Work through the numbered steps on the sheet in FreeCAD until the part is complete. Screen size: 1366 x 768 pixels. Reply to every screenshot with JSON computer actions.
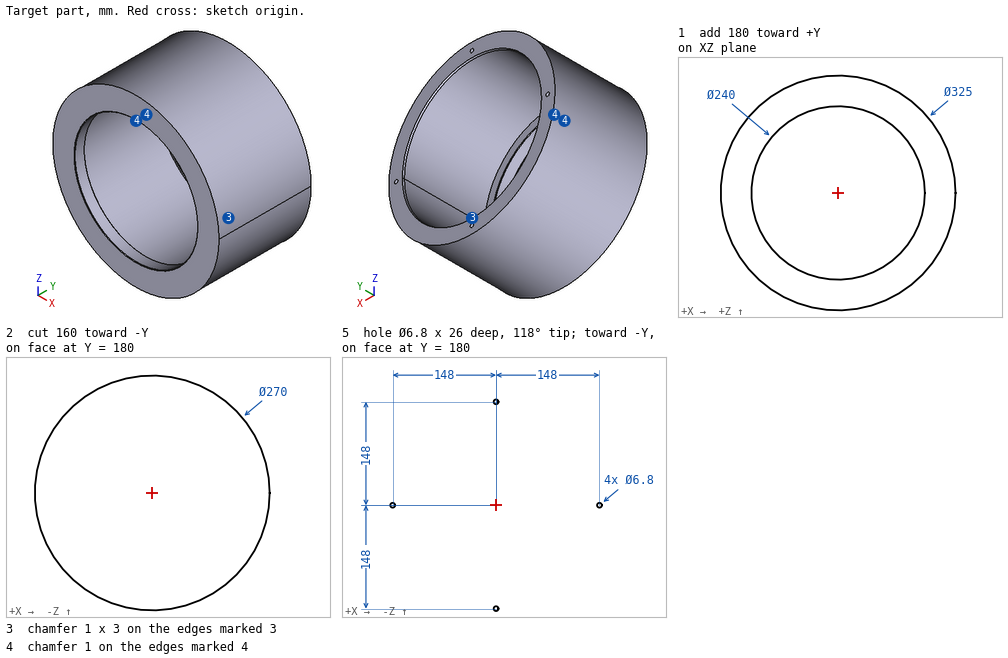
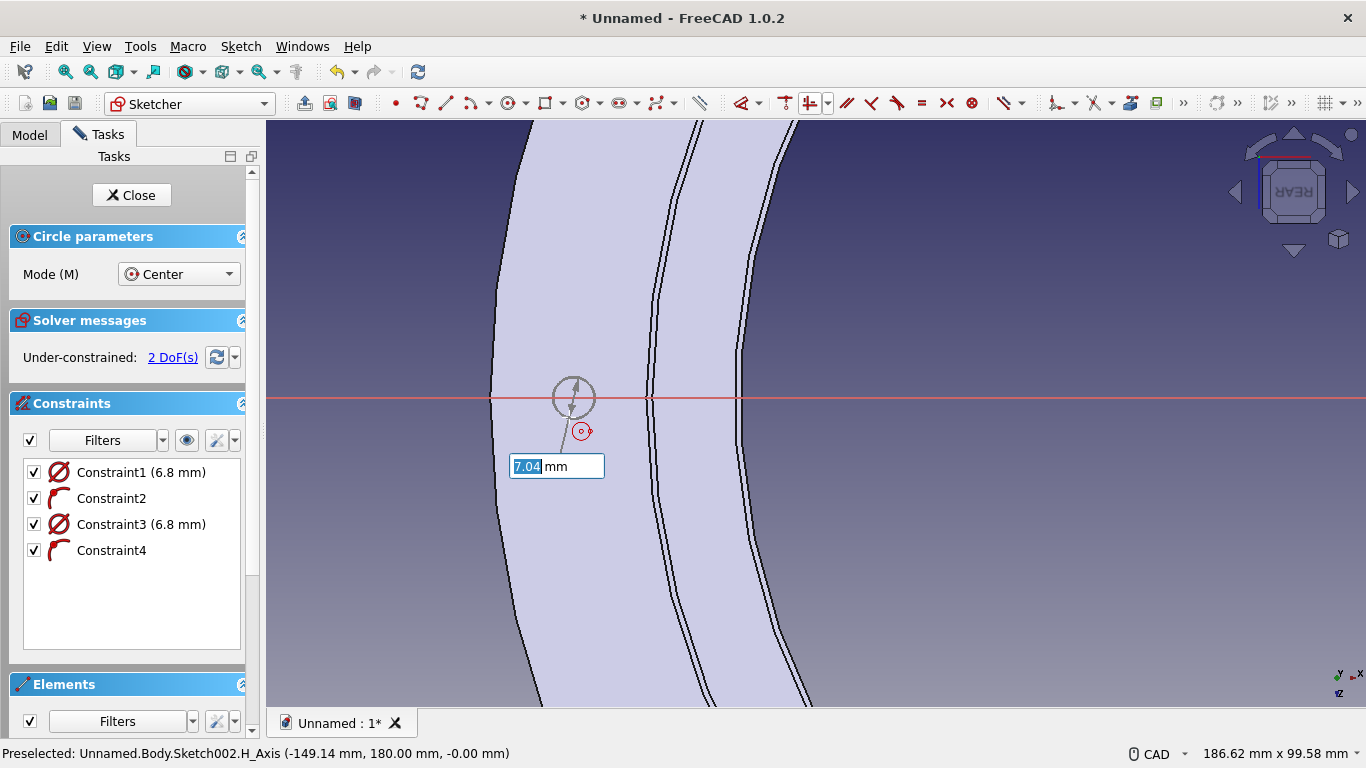
{"action": "type", "text": "6.8"}
{"action": "key", "text": "Return"}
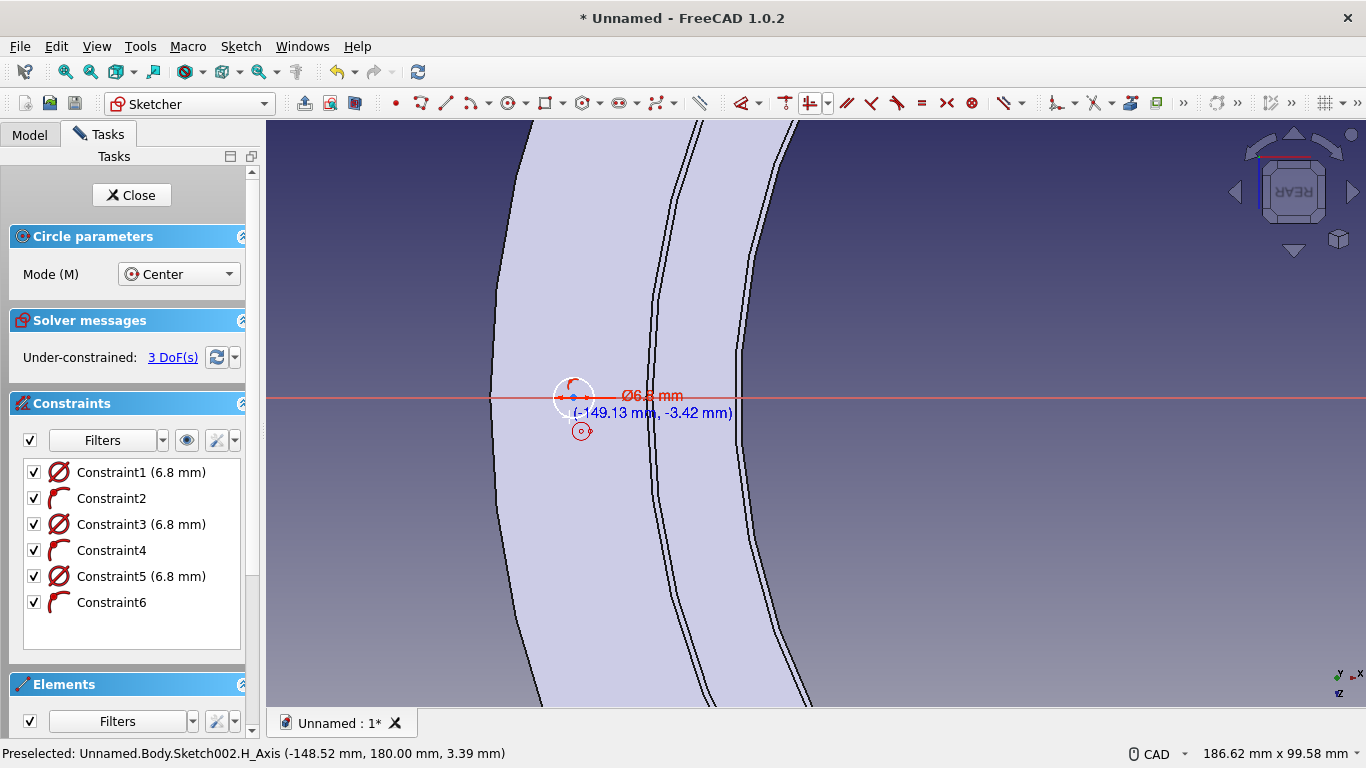
{"action": "scroll", "coordinate": [570, 417], "scroll_direction": "down", "scroll_amount": 8}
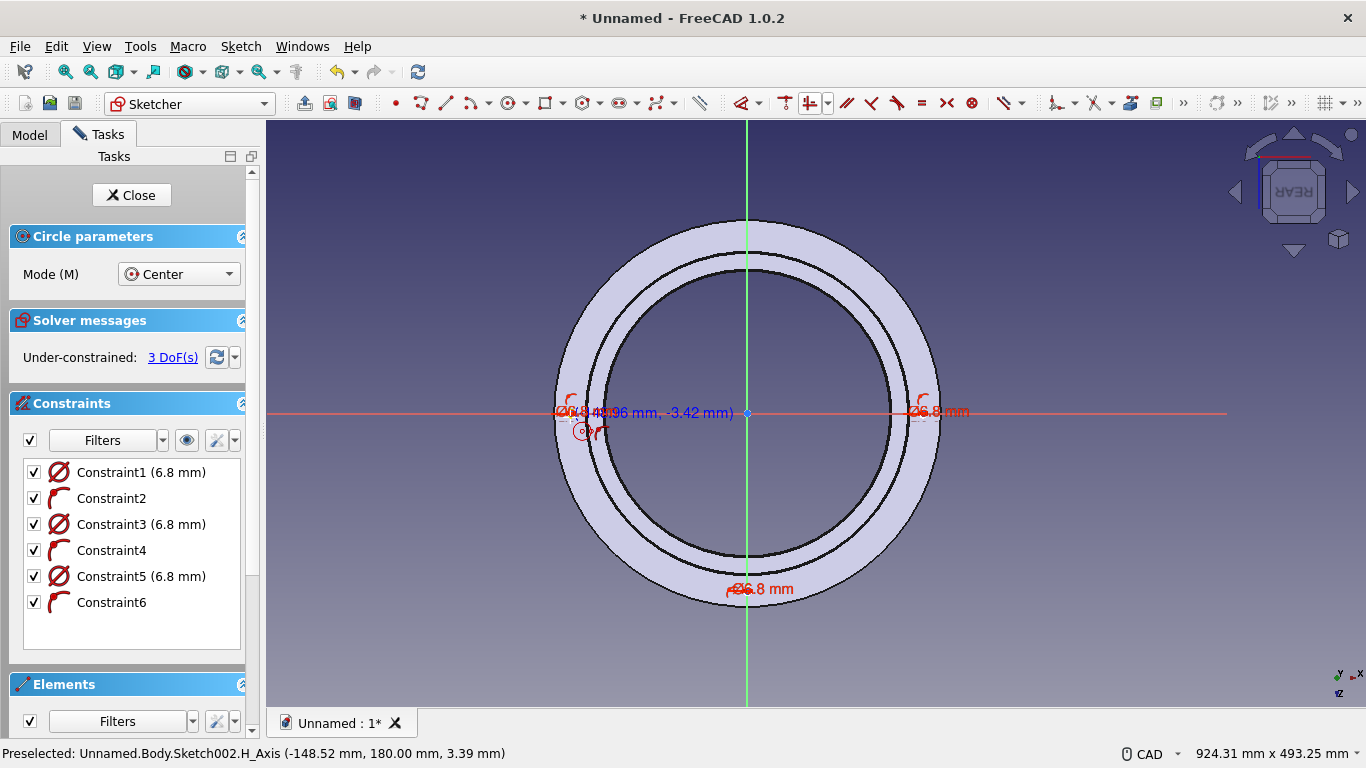
{"action": "scroll", "coordinate": [747, 237], "scroll_direction": "up", "scroll_amount": 9}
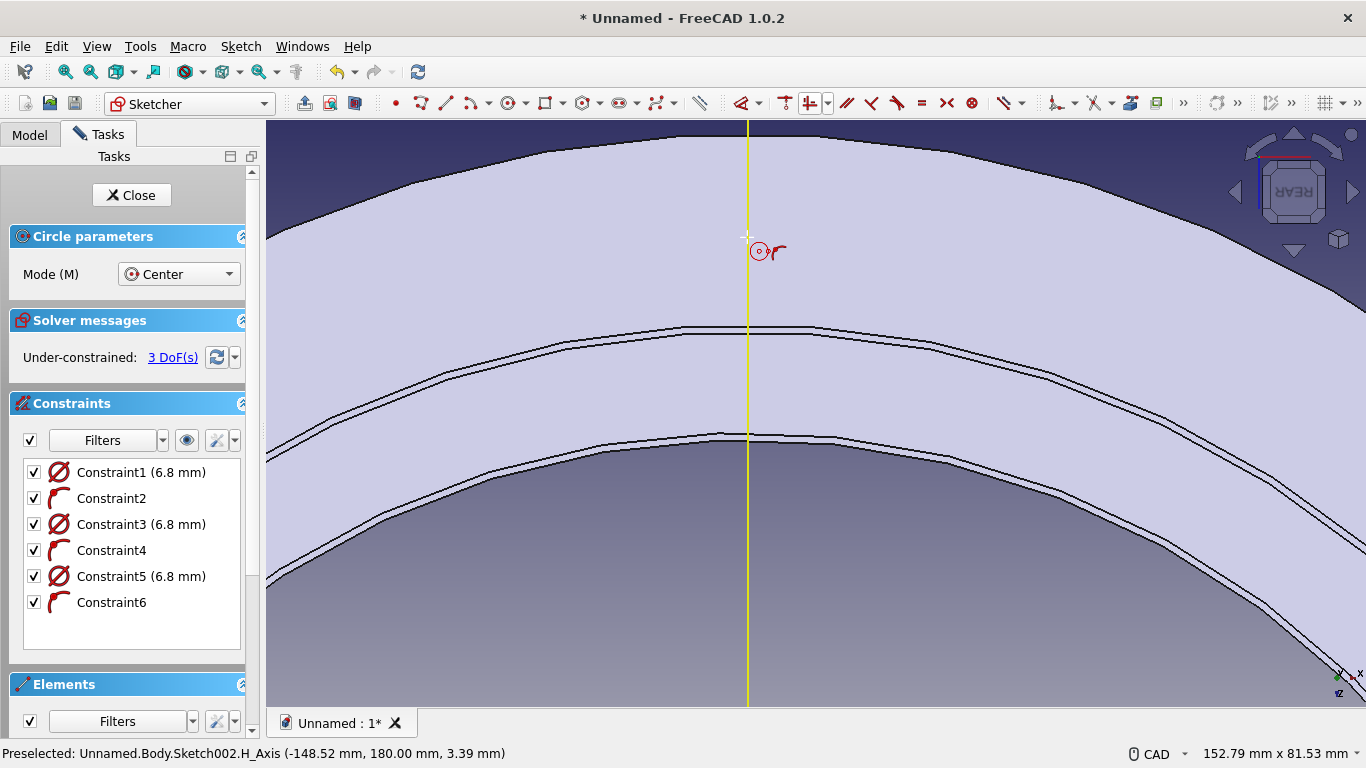
{"action": "scroll", "coordinate": [747, 237], "scroll_direction": "down", "scroll_amount": 9}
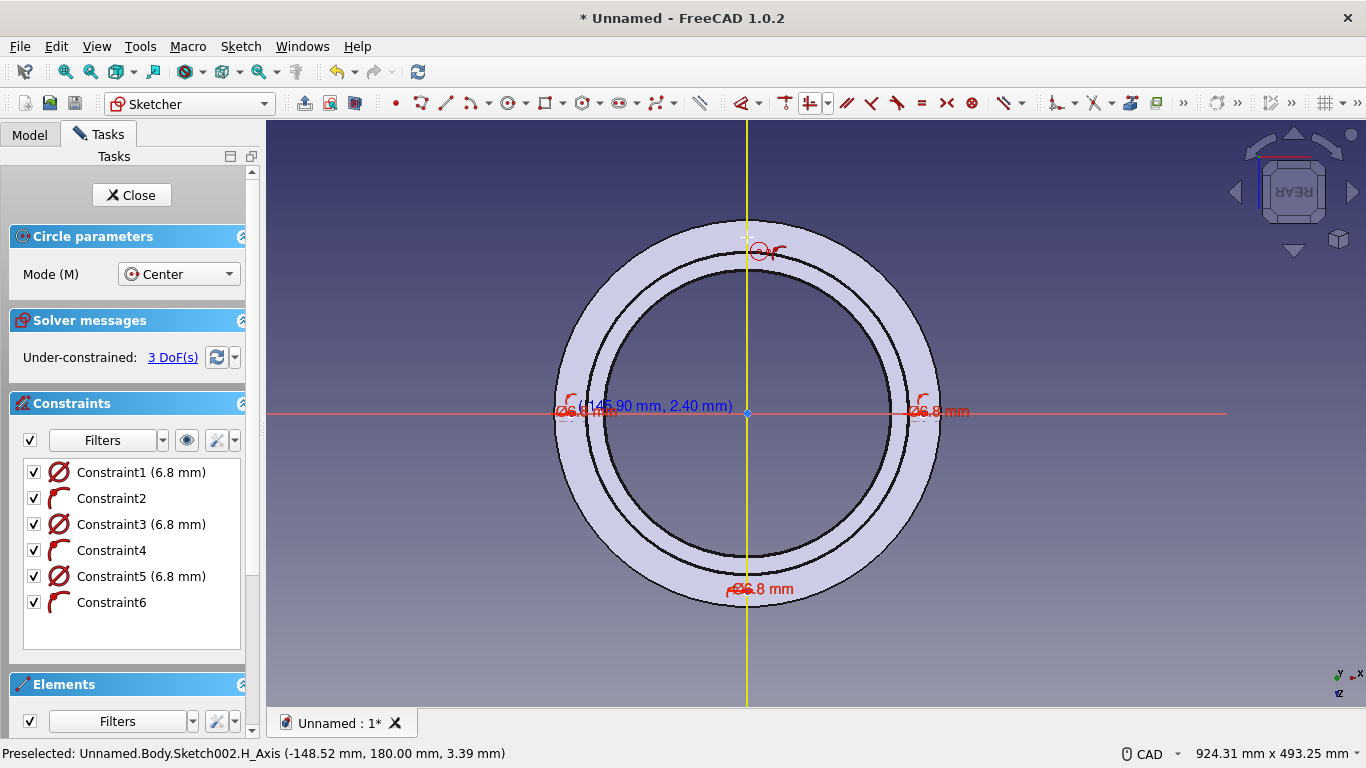
{"action": "left_click", "coordinate": [747, 237]}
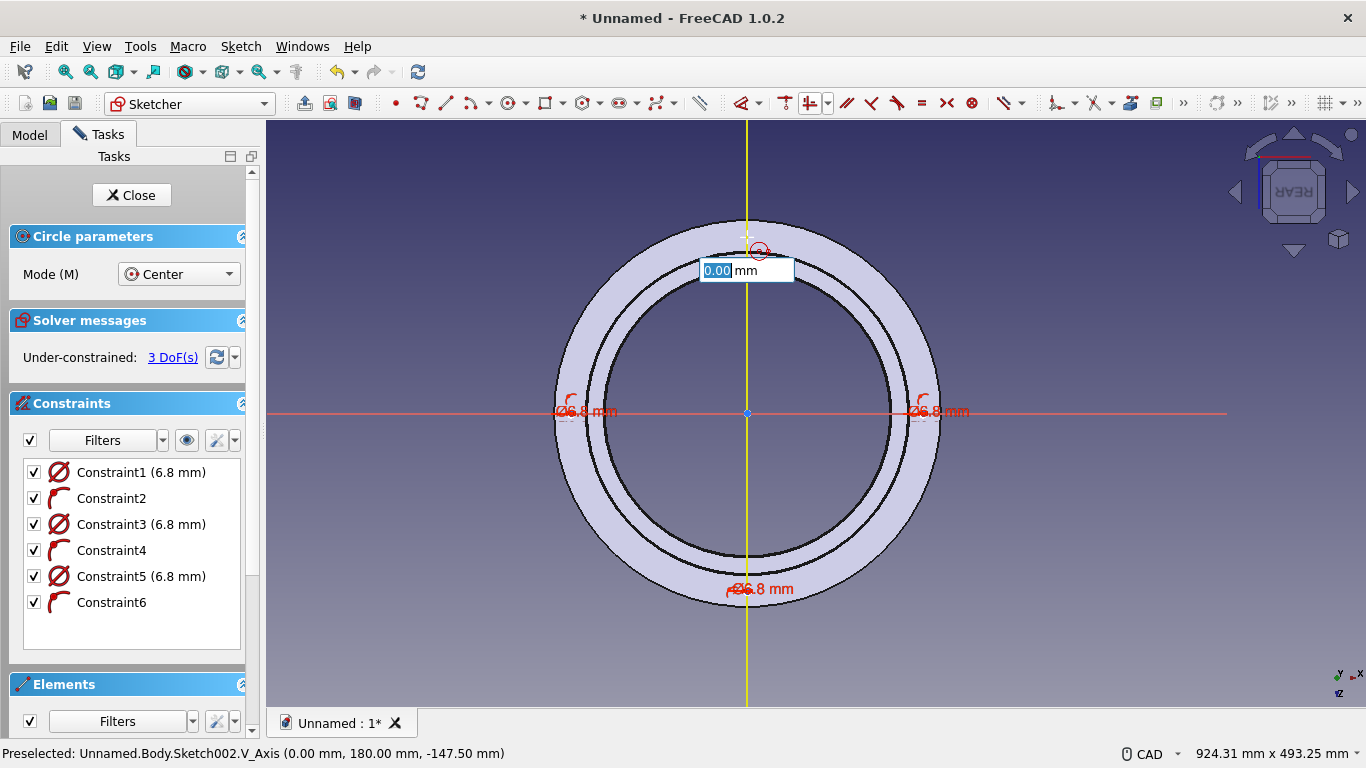
{"action": "scroll", "coordinate": [751, 236], "scroll_direction": "up", "scroll_amount": 8}
{"action": "mouse_move", "coordinate": [751, 235]}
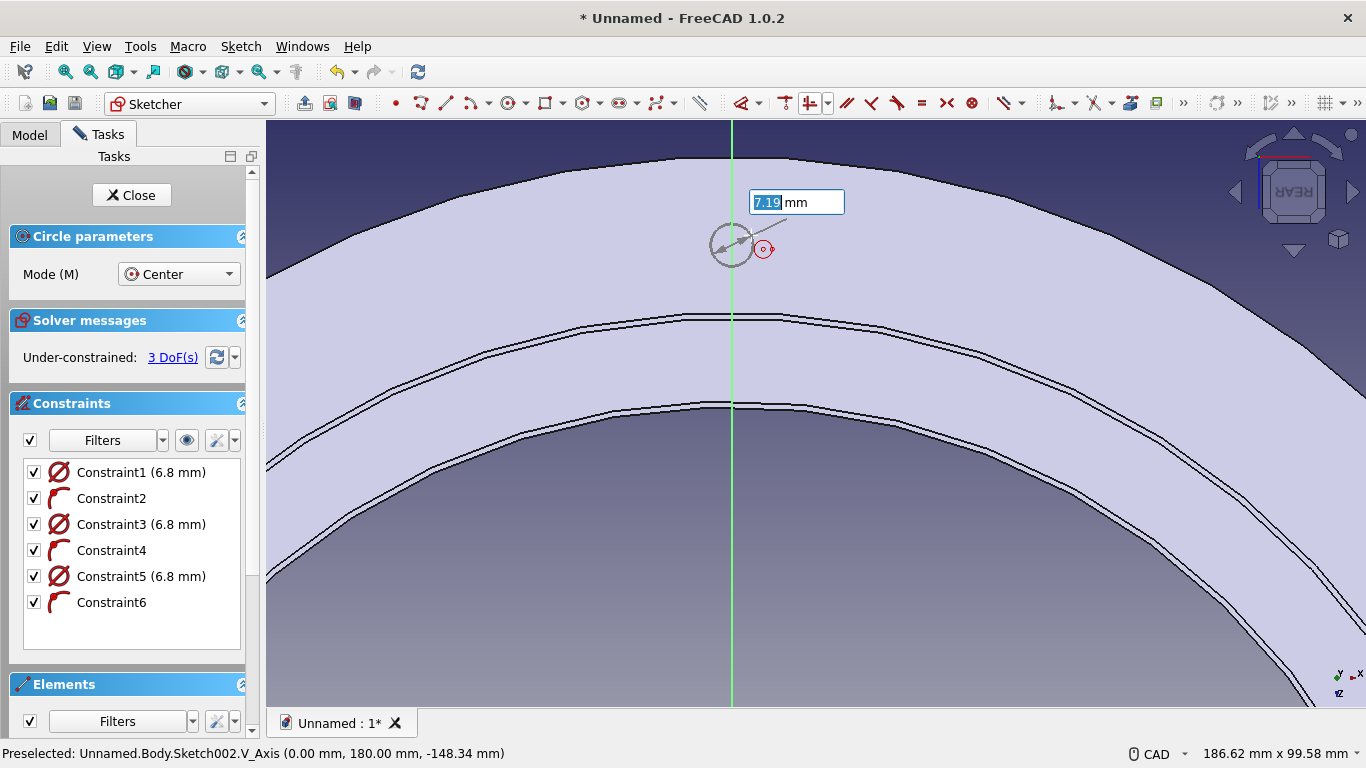
{"action": "type", "text": "6.8"}
{"action": "key", "text": "Return"}
{"action": "key", "text": "Escape"}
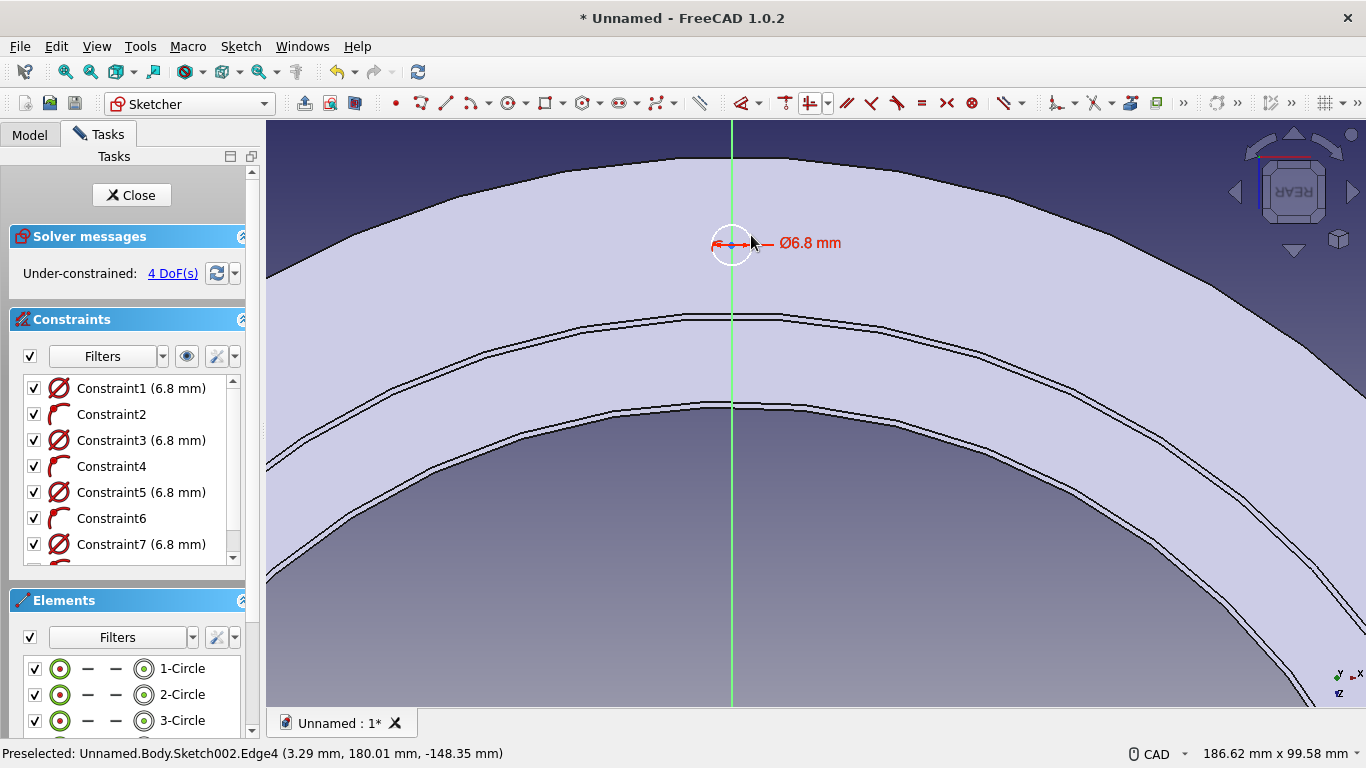
{"action": "key", "text": "d"}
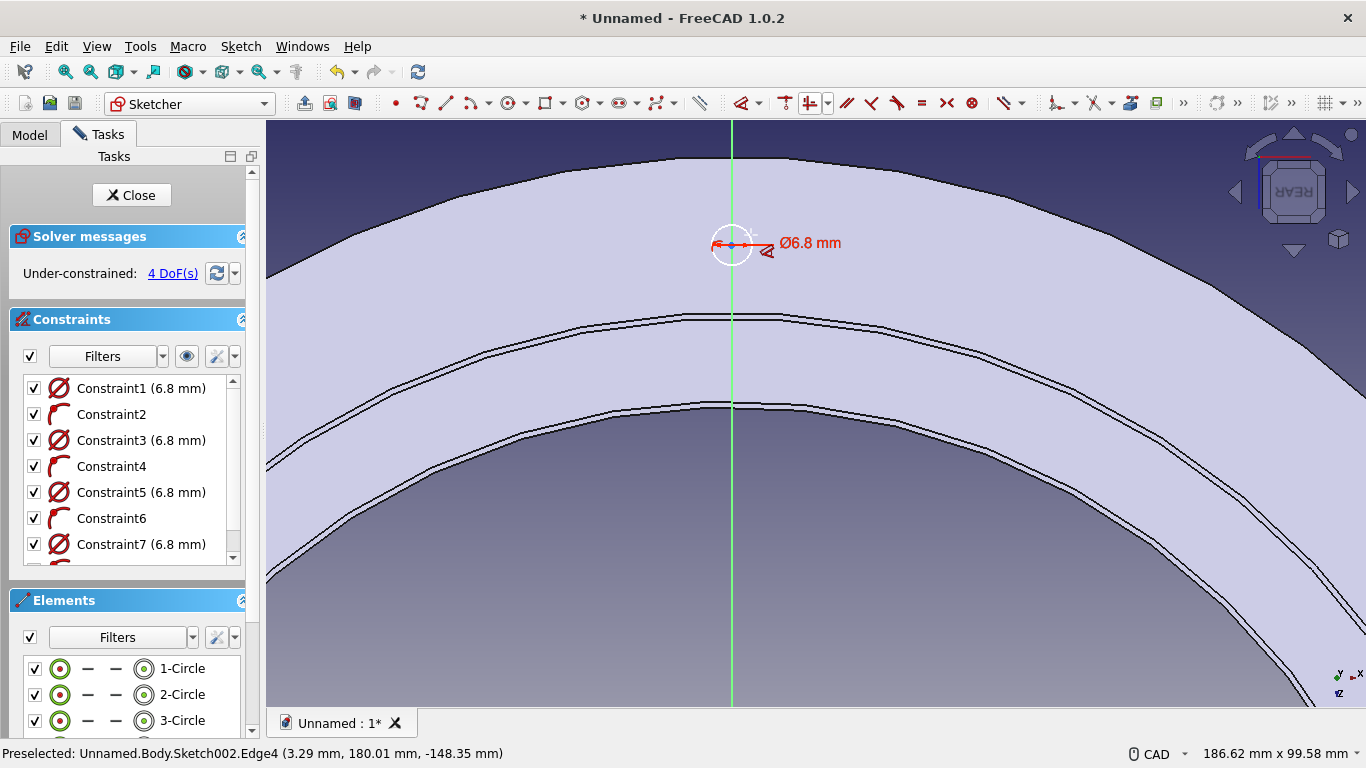
{"action": "scroll", "coordinate": [751, 236], "scroll_direction": "down", "scroll_amount": 8}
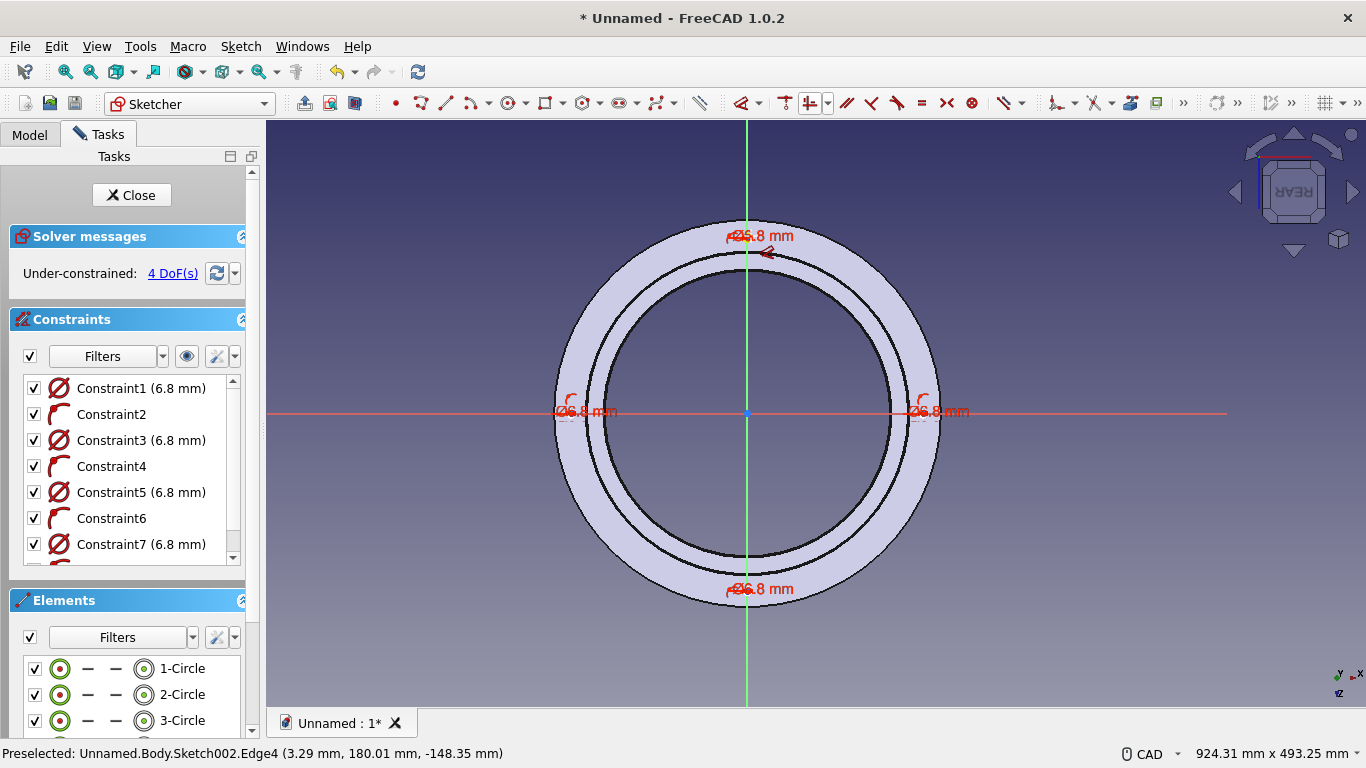
{"action": "left_click", "coordinate": [923, 414]}
{"action": "left_click", "coordinate": [835, 448]}